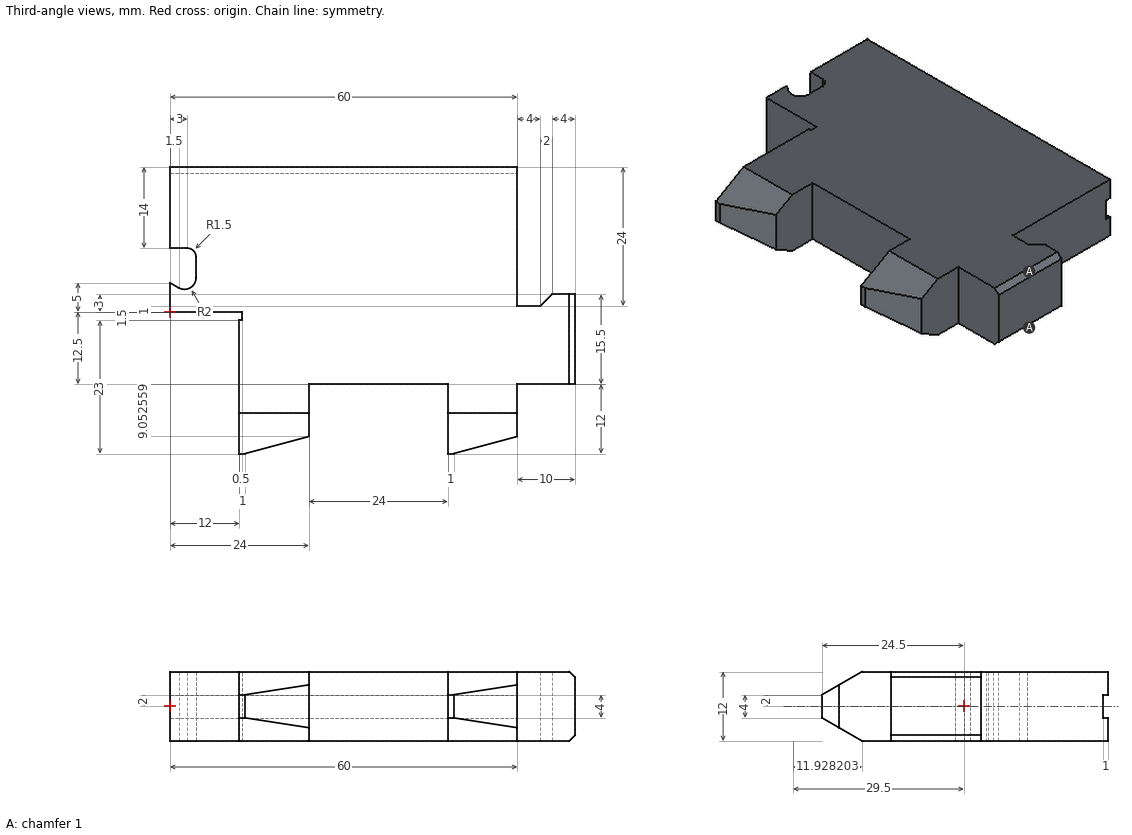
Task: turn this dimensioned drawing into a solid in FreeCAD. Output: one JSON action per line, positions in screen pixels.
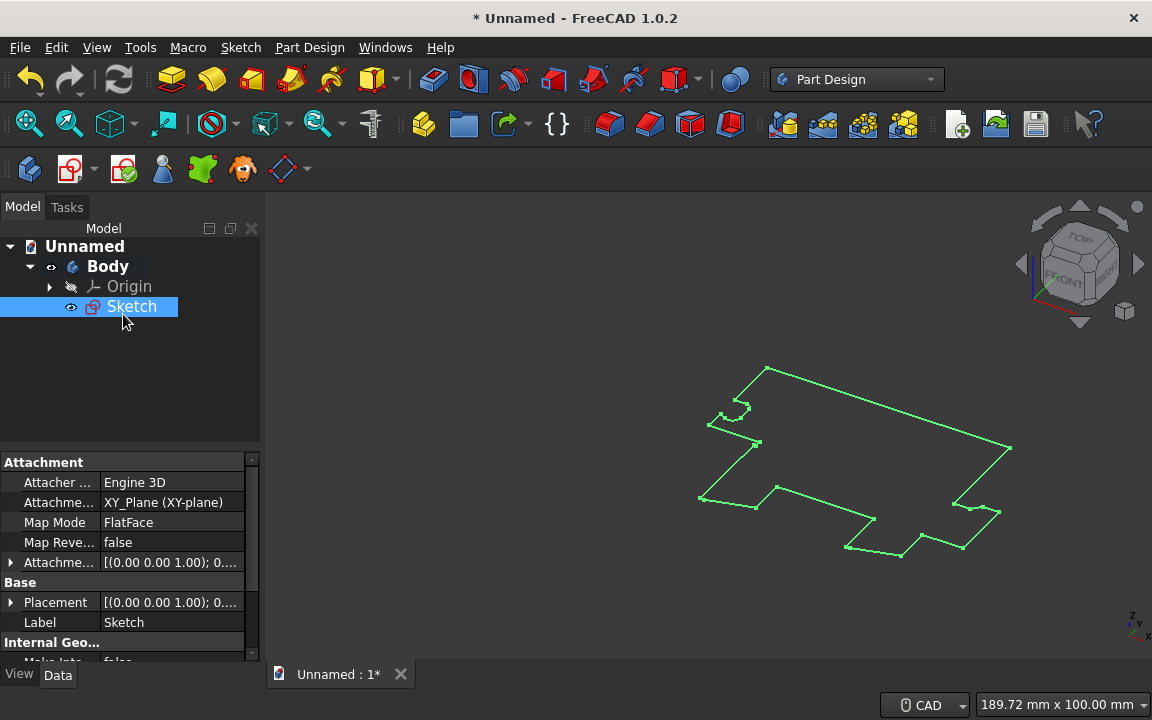
{"action": "left_click", "coordinate": [172, 80]}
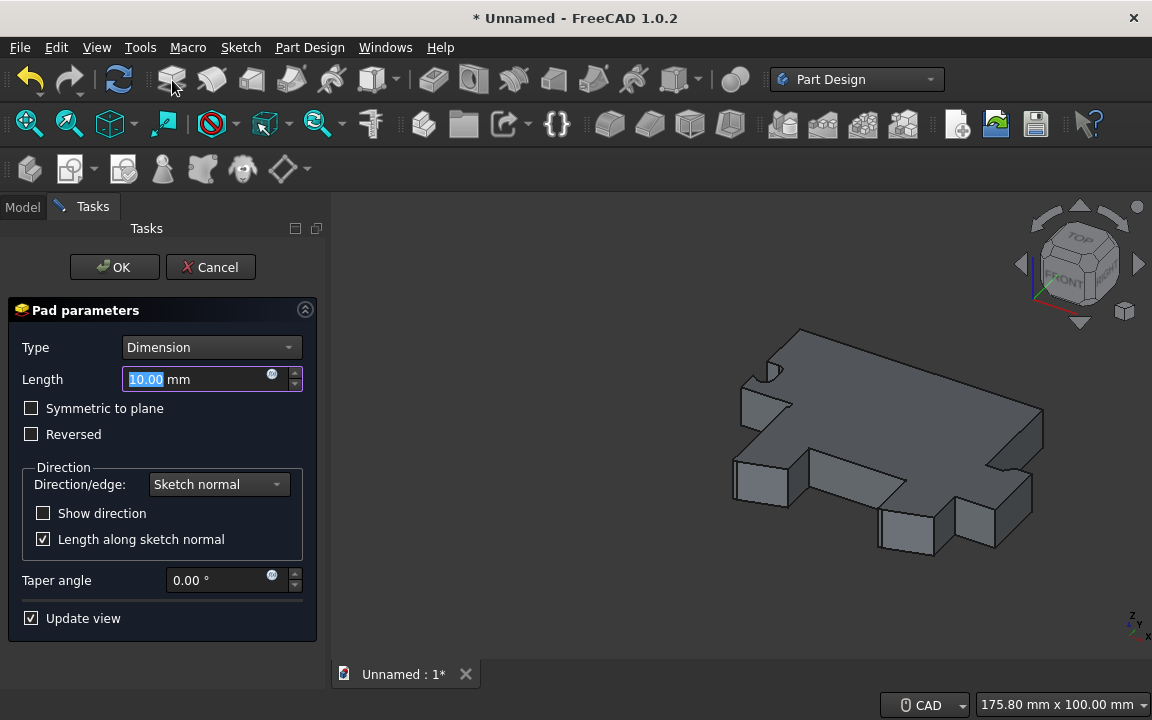
{"action": "type", "text": "12"}
{"action": "key", "text": "Tab"}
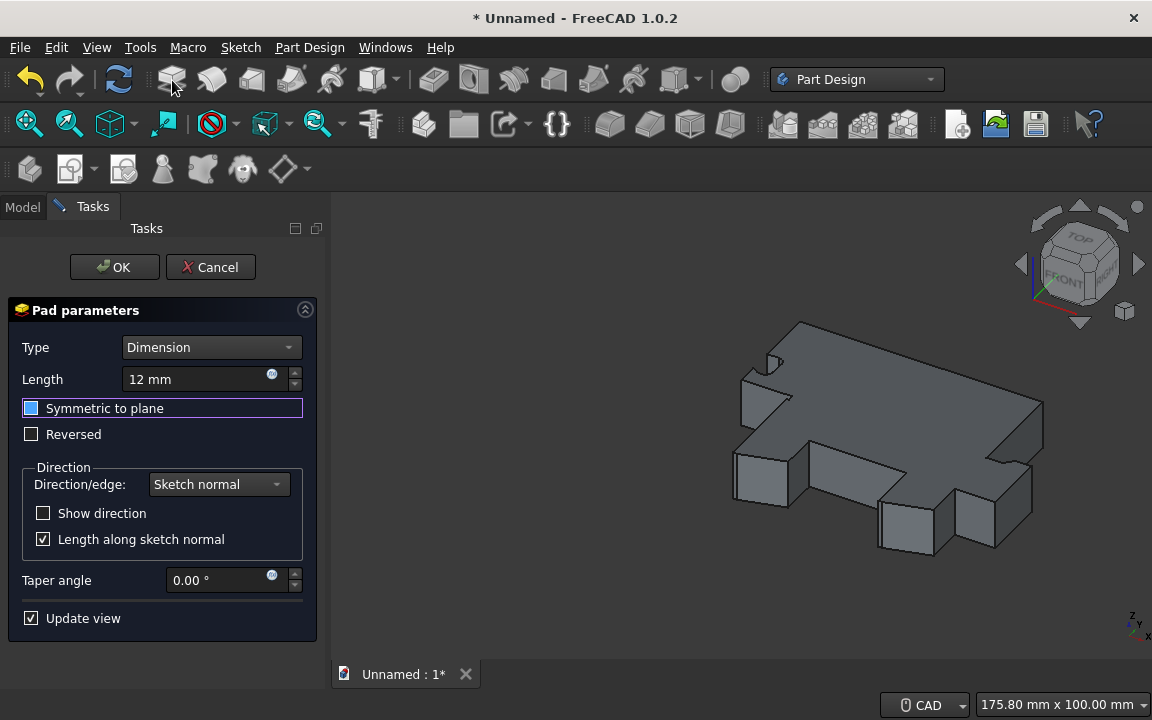
{"action": "left_click", "coordinate": [30, 408]}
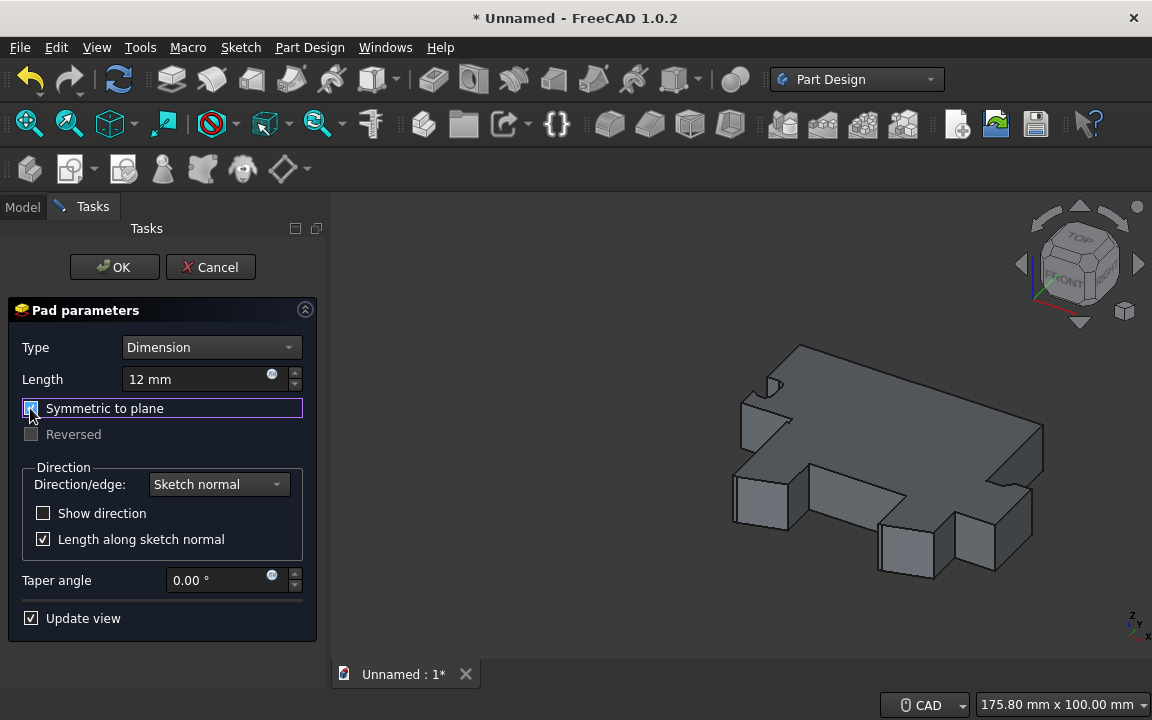
{"action": "left_click", "coordinate": [115, 267]}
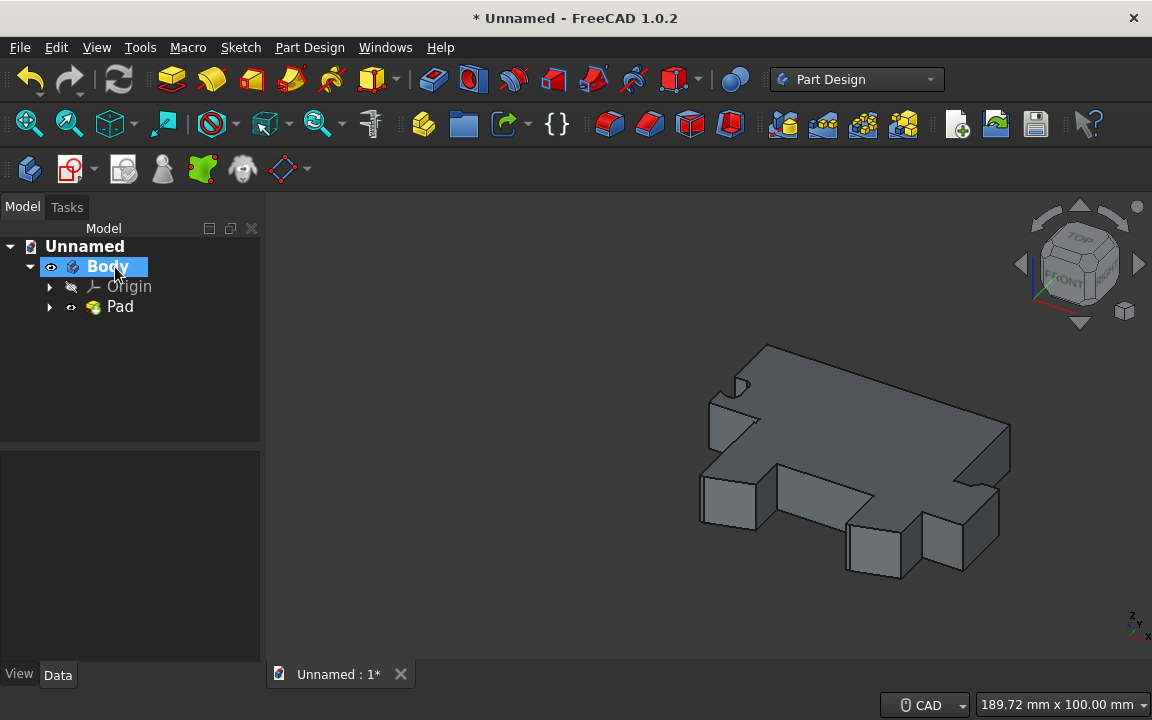
{"action": "key", "text": "6"}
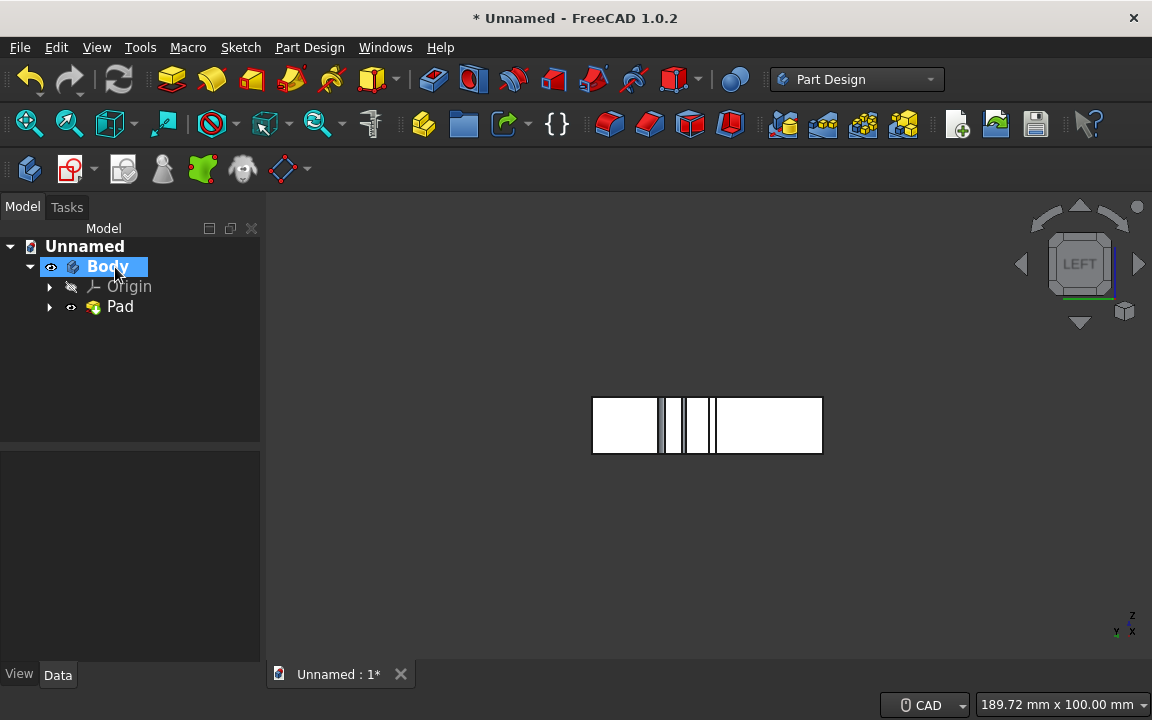
{"action": "left_click", "coordinate": [30, 124]}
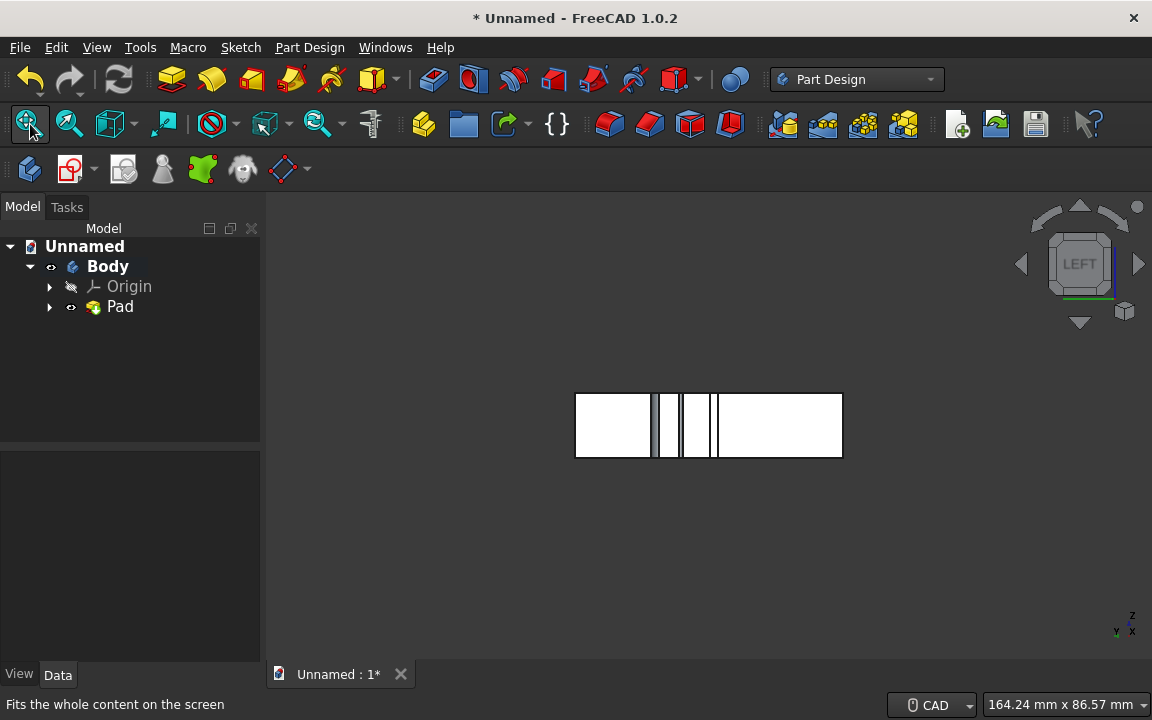
{"action": "left_click", "coordinate": [763, 424]}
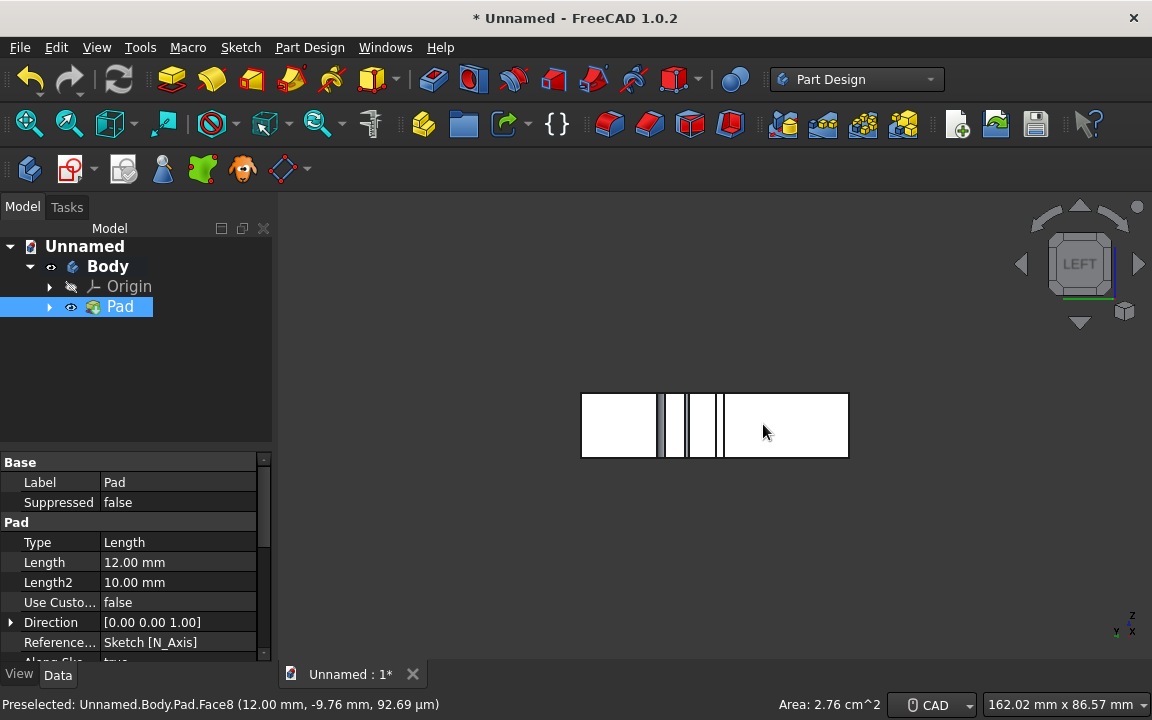
{"action": "left_click", "coordinate": [70, 170]}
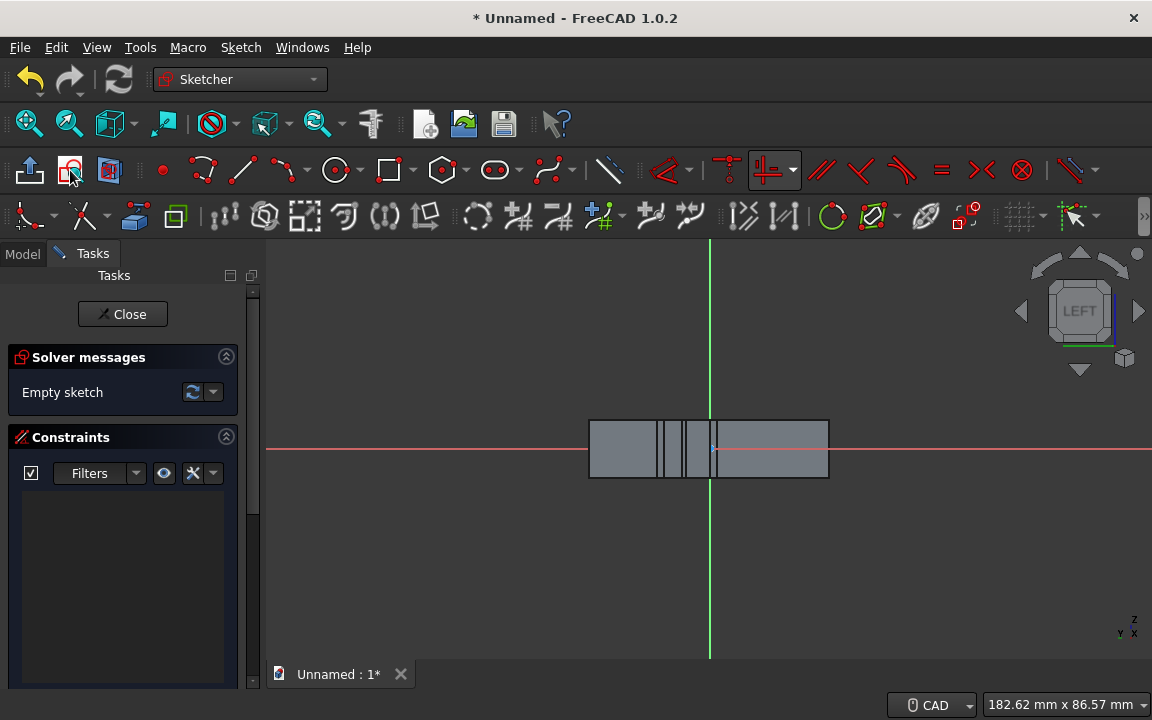
{"action": "left_click", "coordinate": [110, 170]}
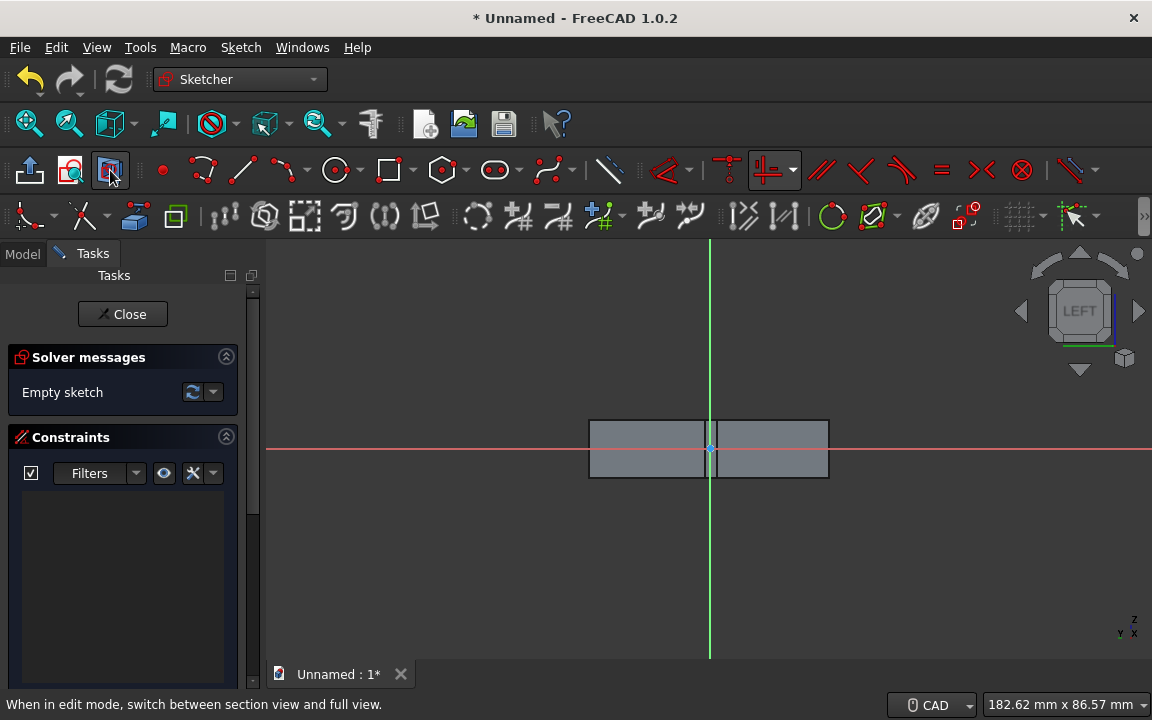
{"action": "scroll", "coordinate": [843, 449], "scroll_direction": "up", "scroll_amount": 6}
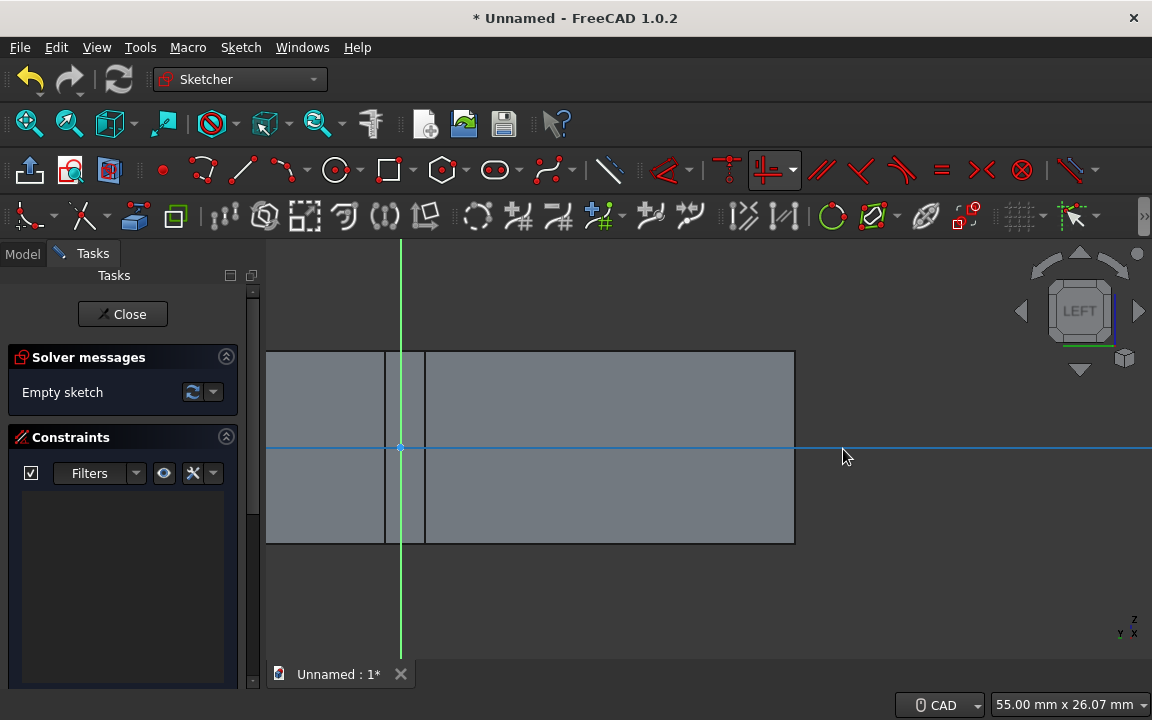
{"action": "left_click", "coordinate": [204, 170]}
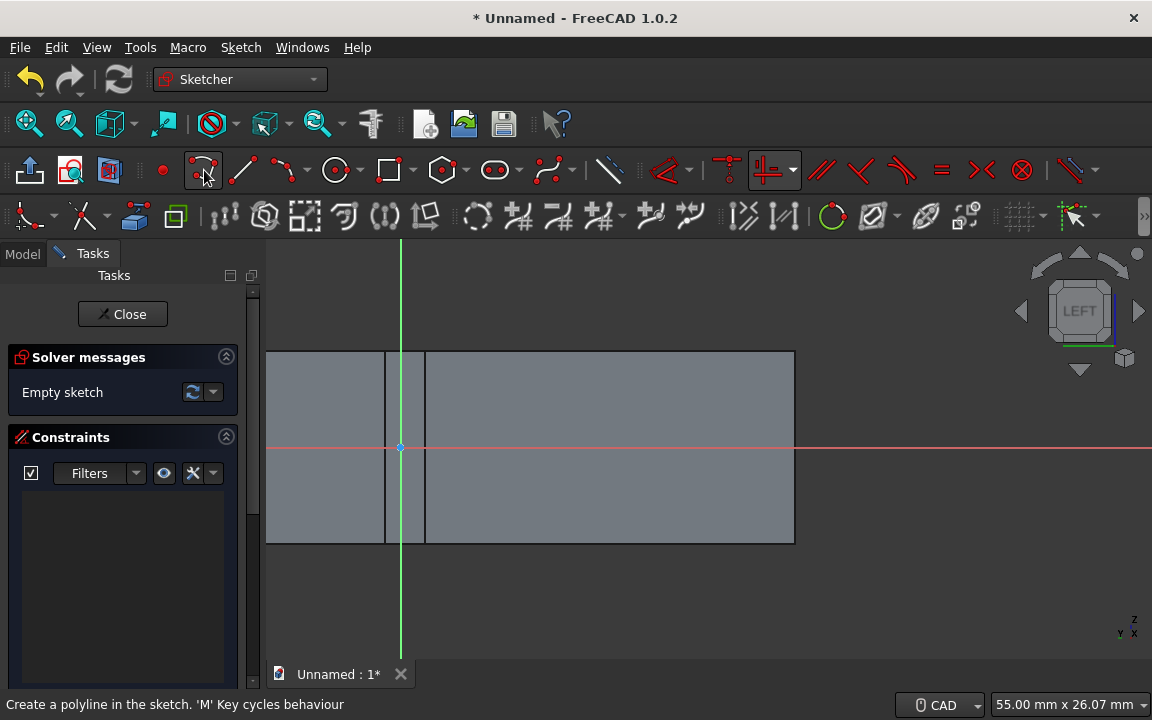
{"action": "left_click", "coordinate": [684, 351]}
{"action": "left_click", "coordinate": [795, 416]}
{"action": "left_click", "coordinate": [795, 480]}
{"action": "left_click", "coordinate": [684, 544]}
{"action": "left_click", "coordinate": [876, 544]}
{"action": "left_click", "coordinate": [876, 351]}
{"action": "left_click", "coordinate": [684, 352]}
{"action": "key", "text": "Escape"}
{"action": "key", "text": "Escape"}